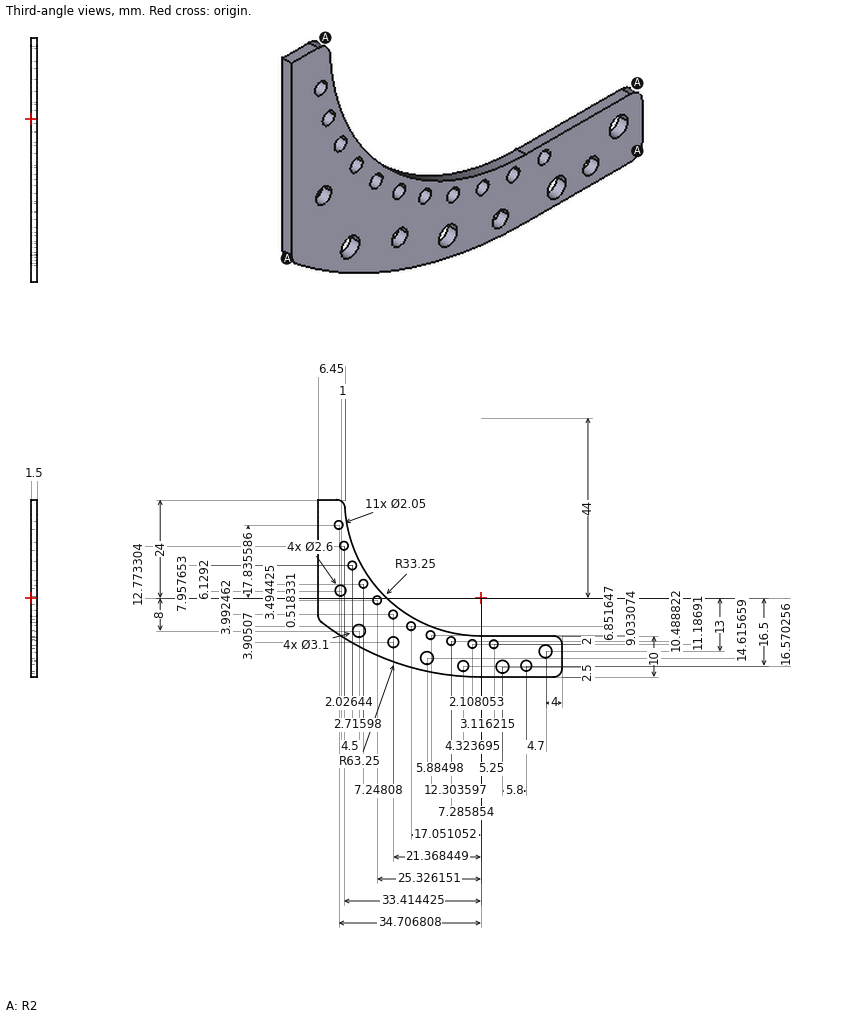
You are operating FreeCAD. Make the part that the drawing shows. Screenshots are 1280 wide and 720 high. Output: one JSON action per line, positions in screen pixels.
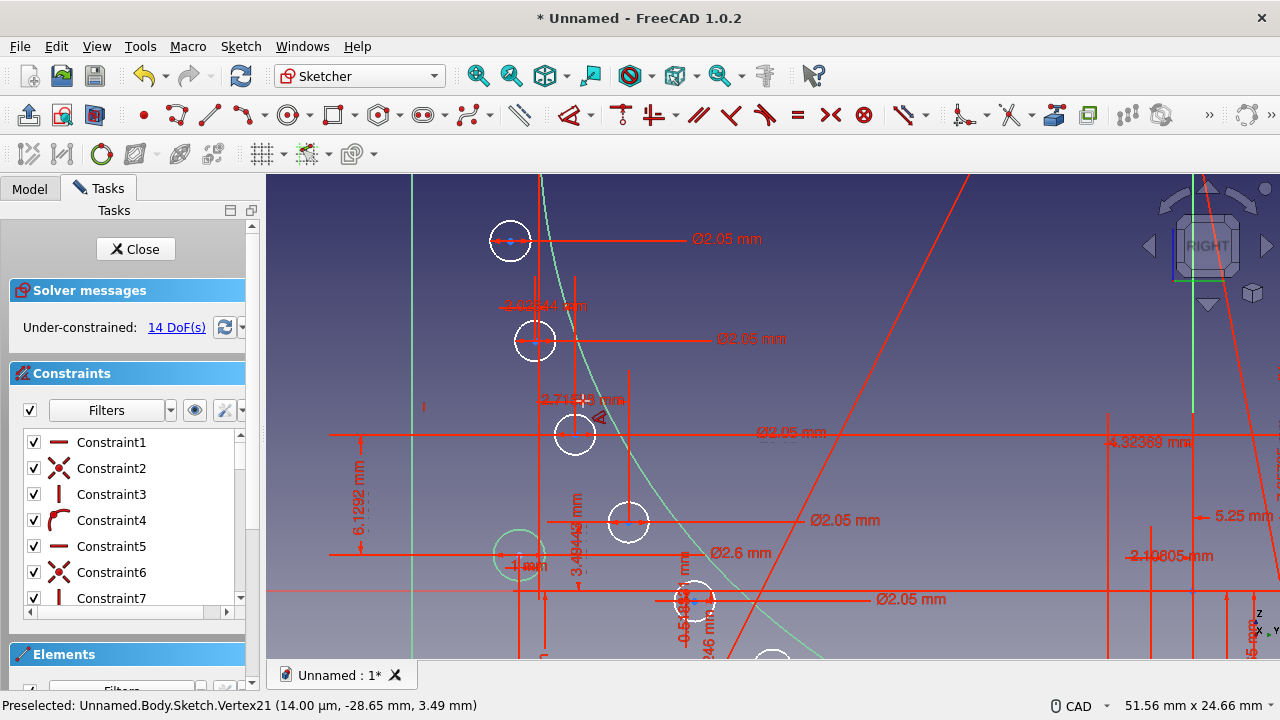
{"action": "left_click", "coordinate": [629, 522]}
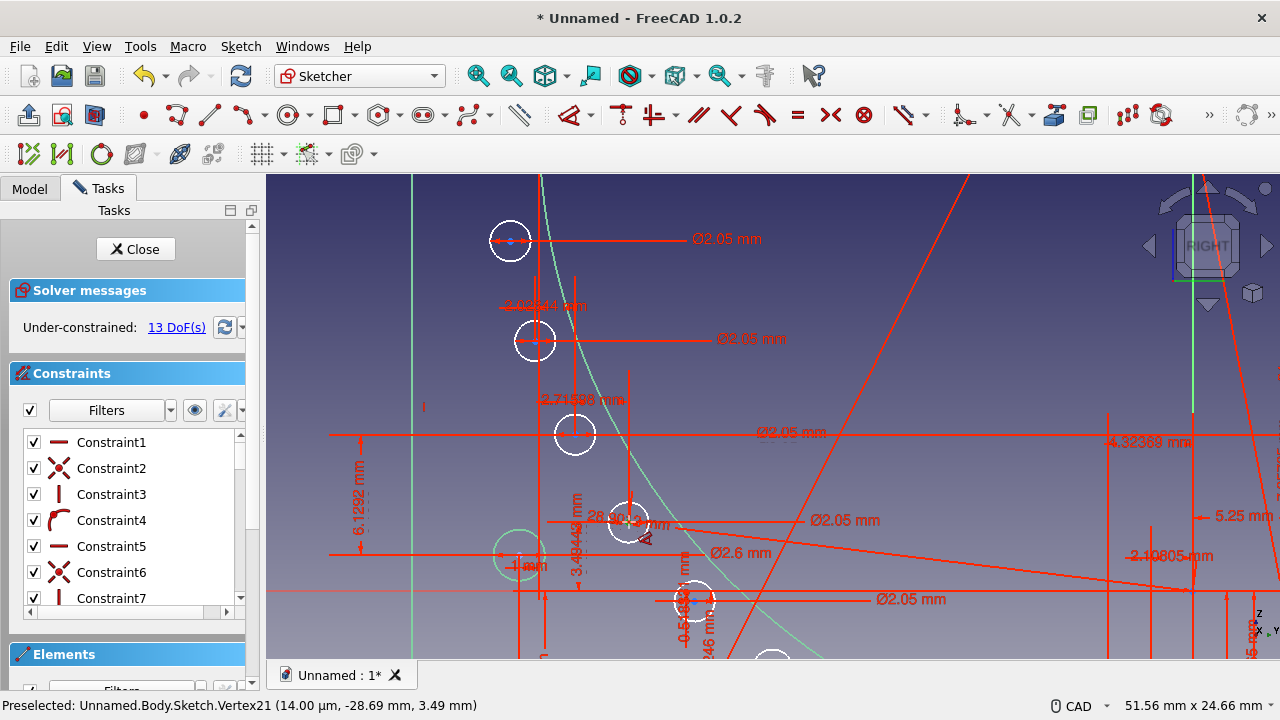
{"action": "scroll", "coordinate": [534, 342], "scroll_direction": "down", "scroll_amount": 5}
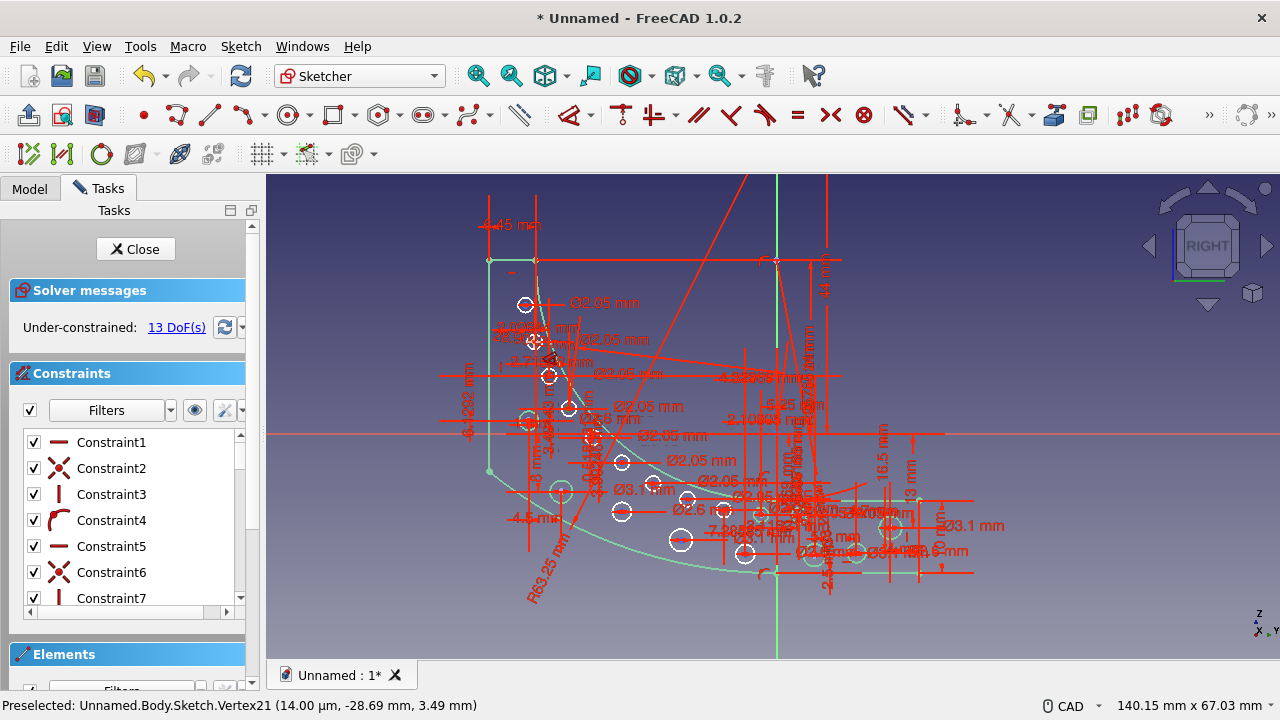
{"action": "left_click", "coordinate": [622, 463]}
{"action": "left_click", "coordinate": [595, 497]}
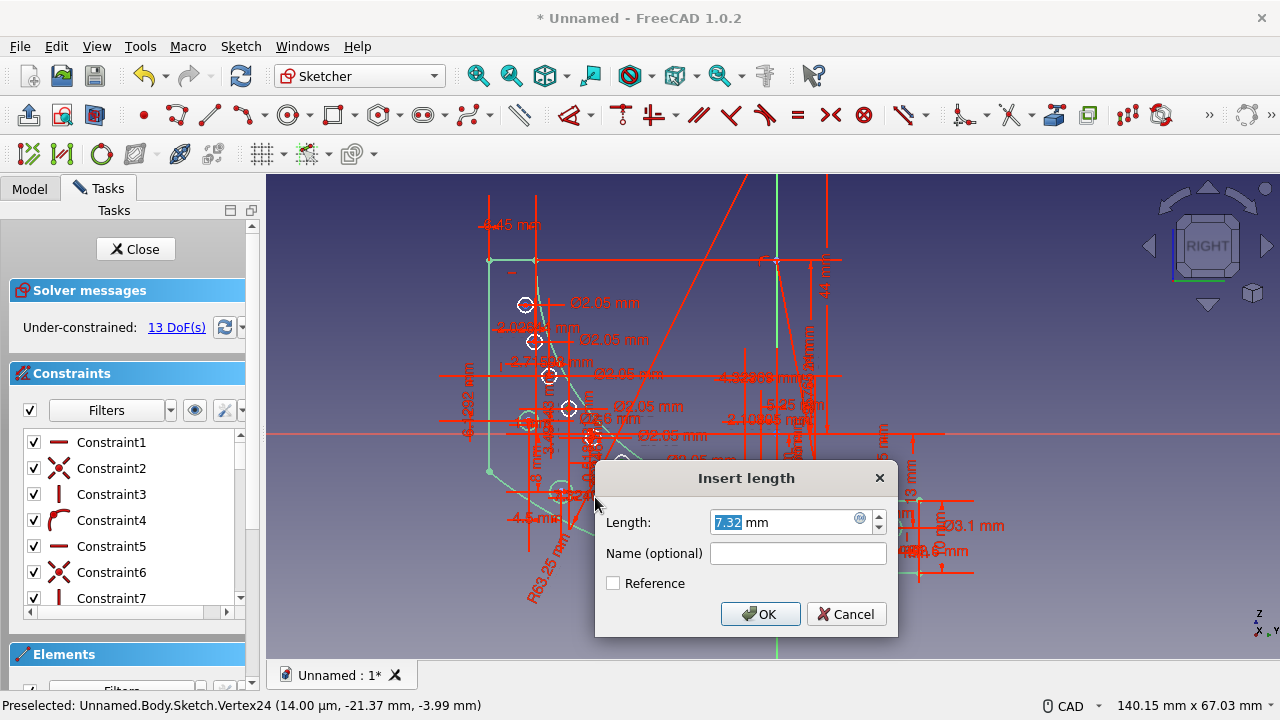
{"action": "type", "text": "7.24808"}
{"action": "key", "text": "Return"}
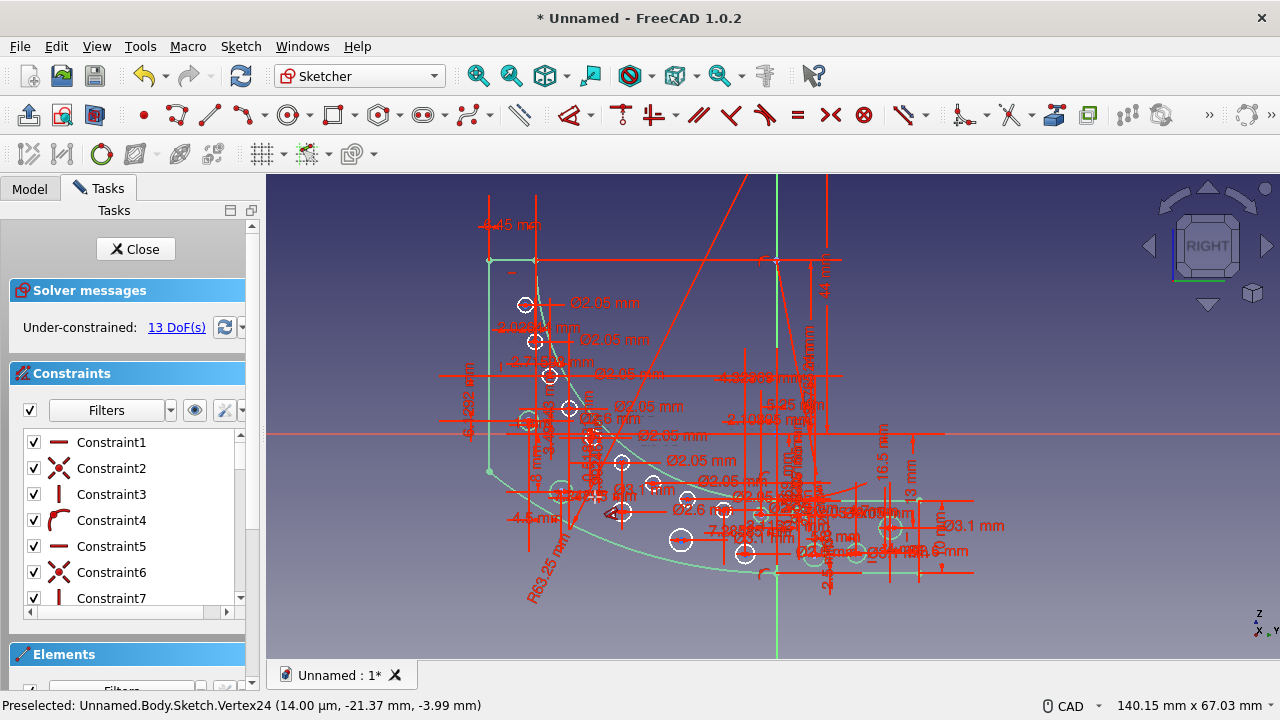
{"action": "scroll", "coordinate": [653, 483], "scroll_direction": "up", "scroll_amount": 2}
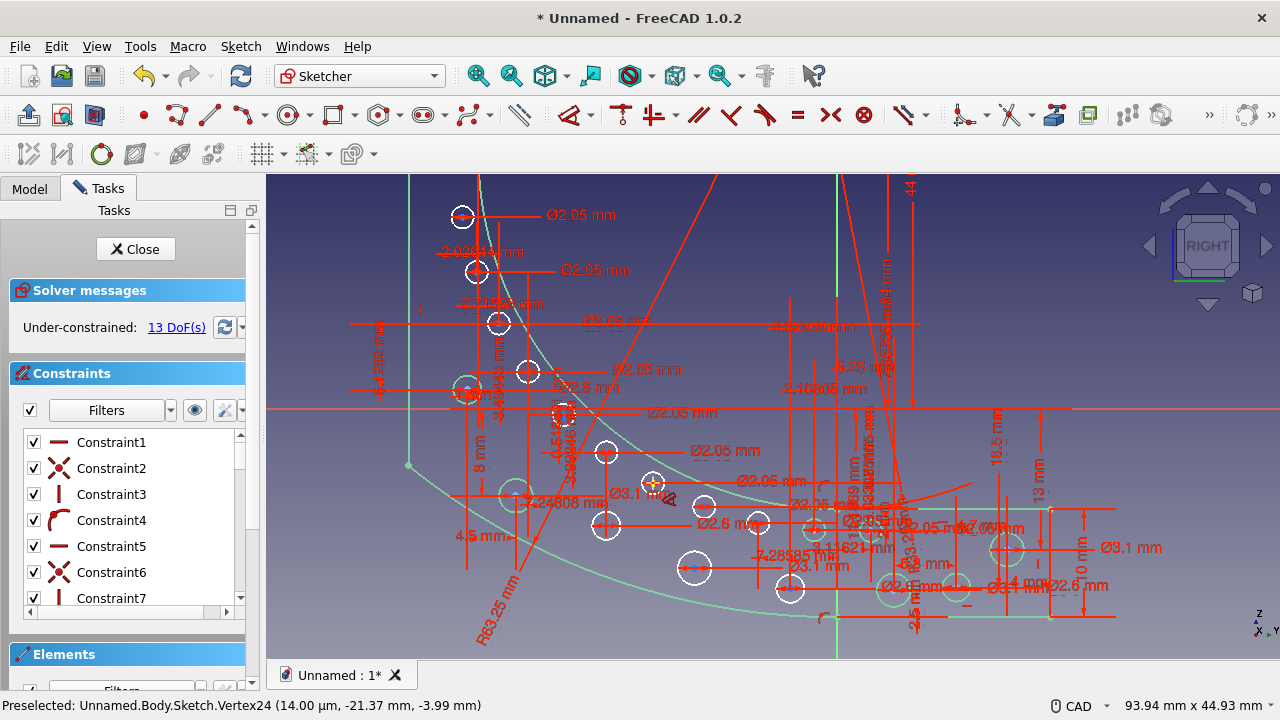
{"action": "left_click", "coordinate": [653, 483]}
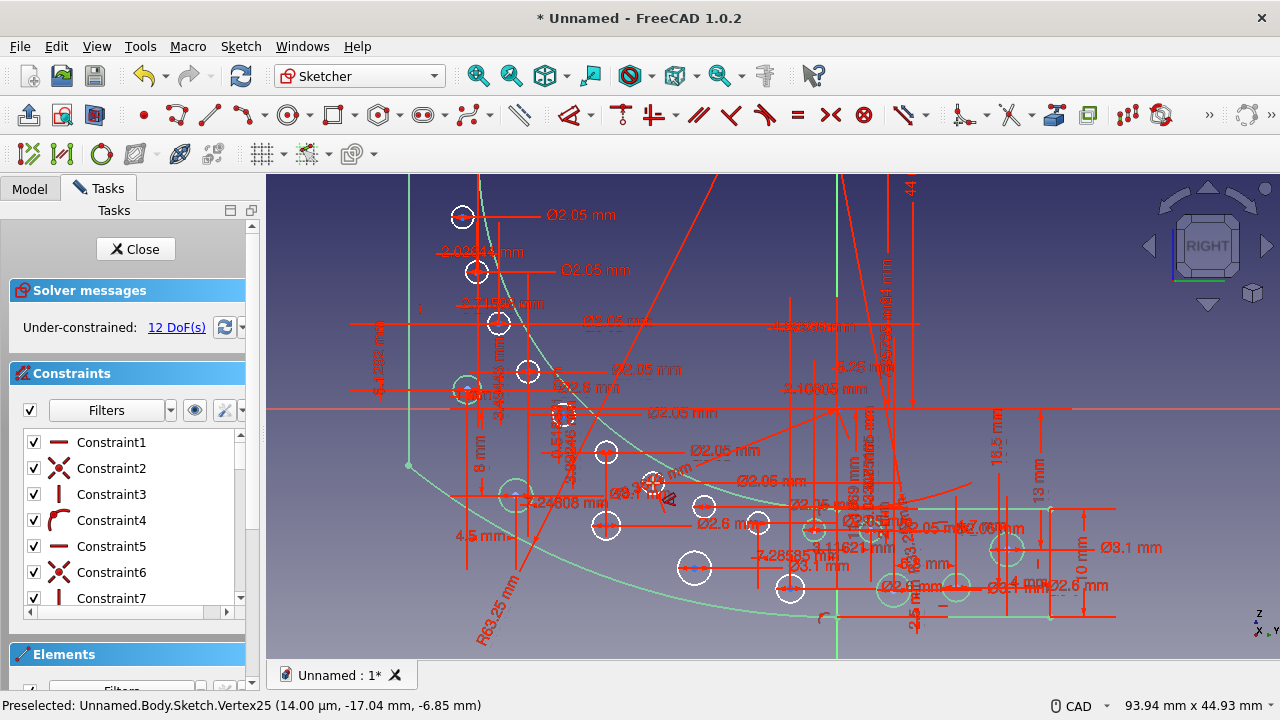
{"action": "left_click", "coordinate": [606, 526]}
{"action": "left_click", "coordinate": [735, 514]}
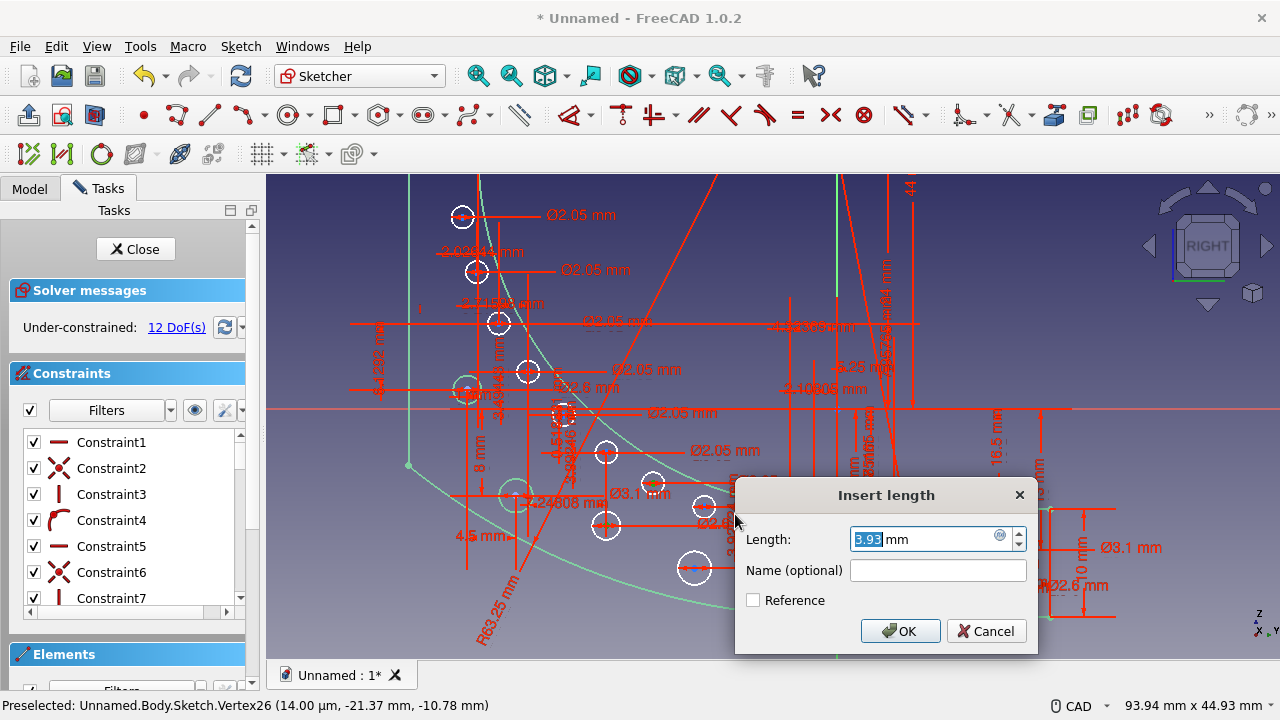
{"action": "type", "text": "3.90507"}
{"action": "key", "text": "Return"}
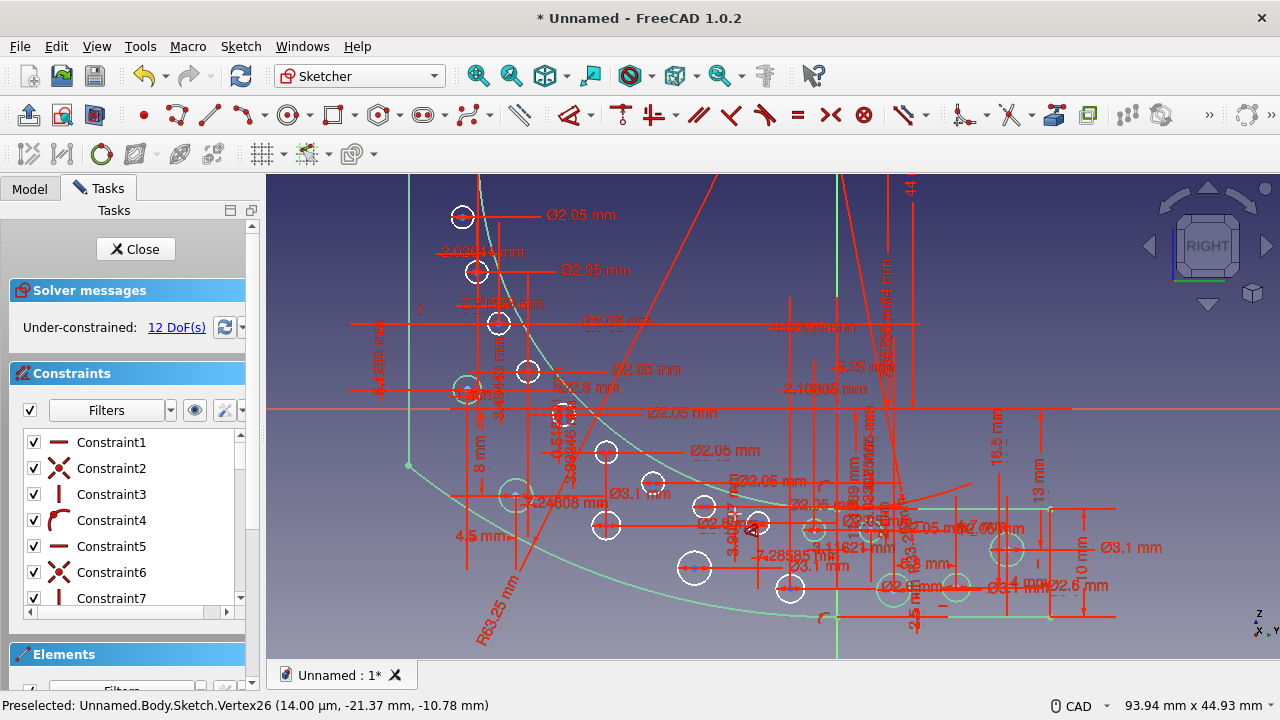
{"action": "left_click", "coordinate": [695, 568]}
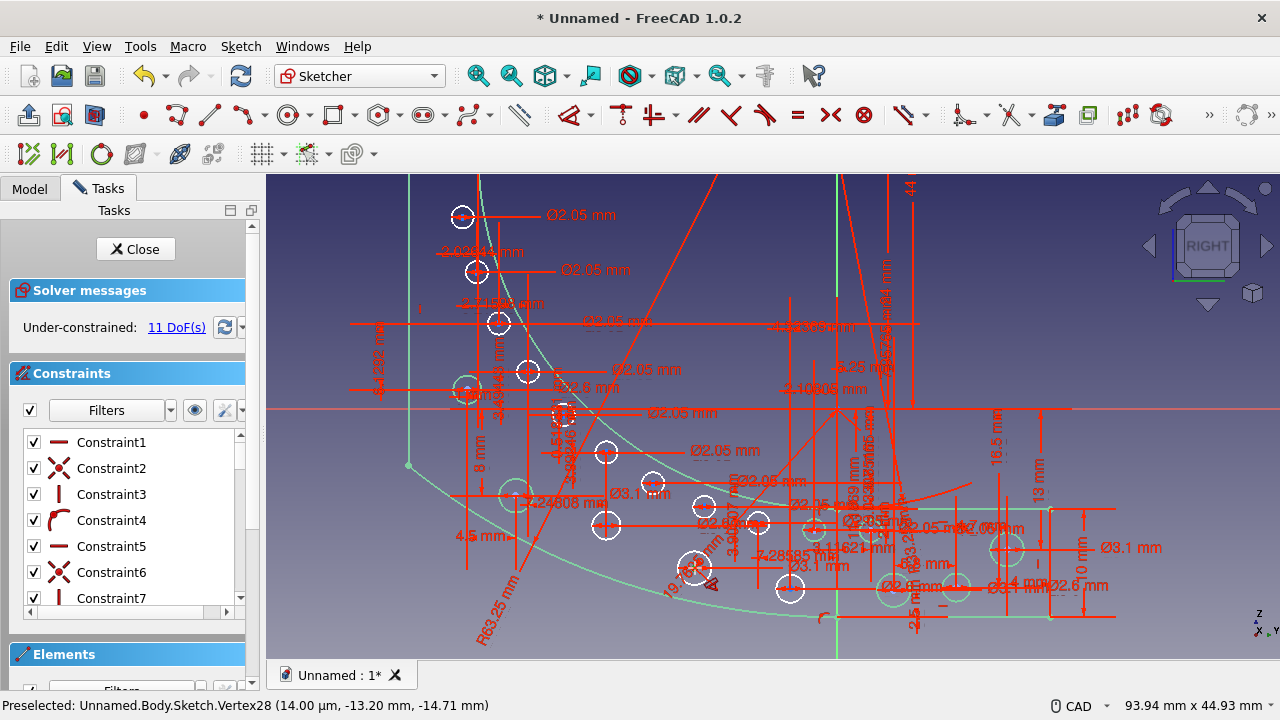
{"action": "left_click", "coordinate": [758, 523]}
{"action": "left_click", "coordinate": [727, 626]}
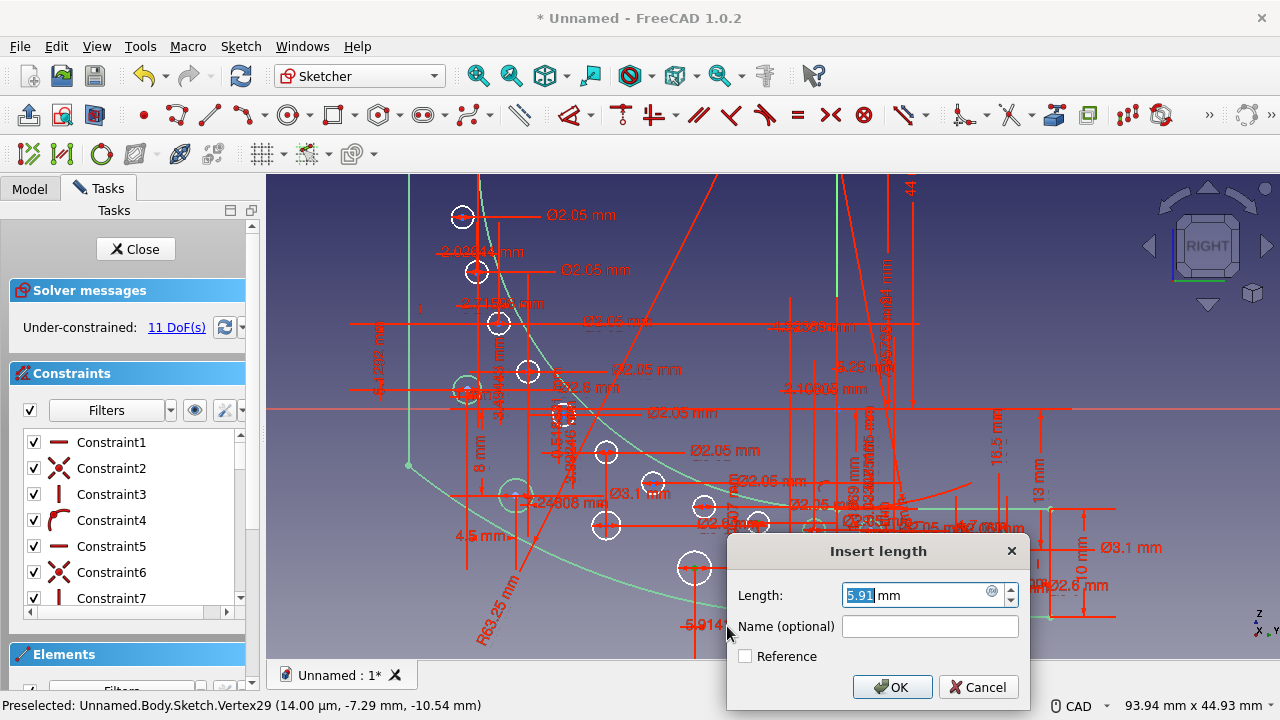
{"action": "type", "text": "5.88498"}
{"action": "key", "text": "Return"}